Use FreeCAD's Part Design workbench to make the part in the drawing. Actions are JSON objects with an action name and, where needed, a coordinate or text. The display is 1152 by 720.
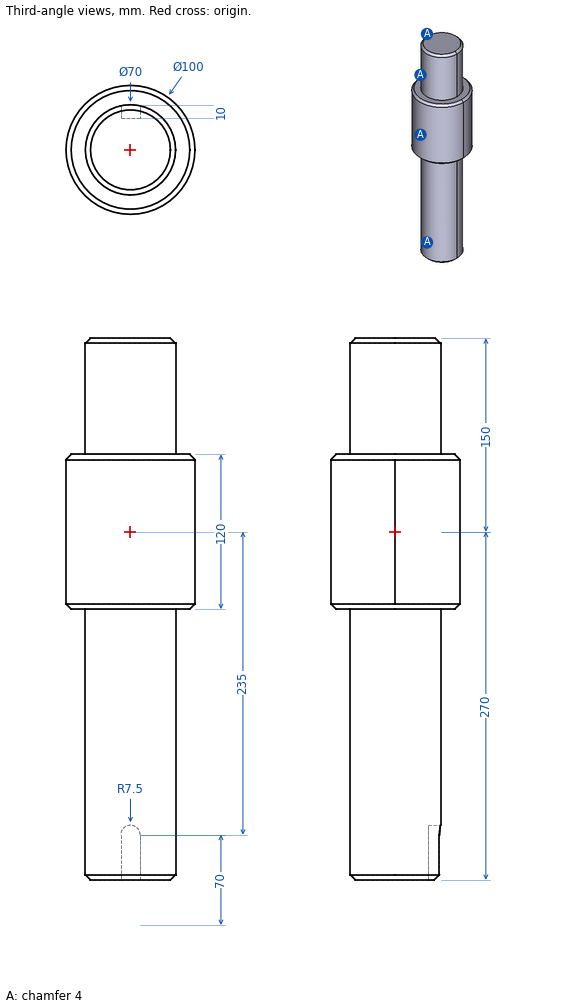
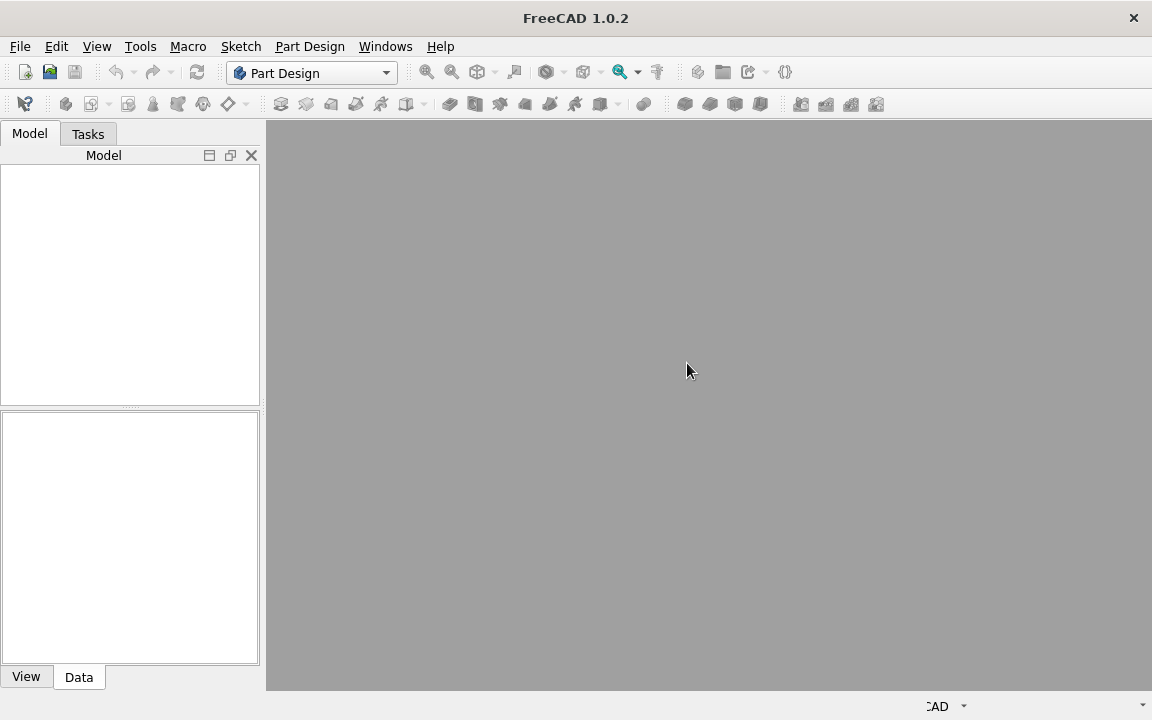
{"action": "left_click", "coordinate": [25, 72]}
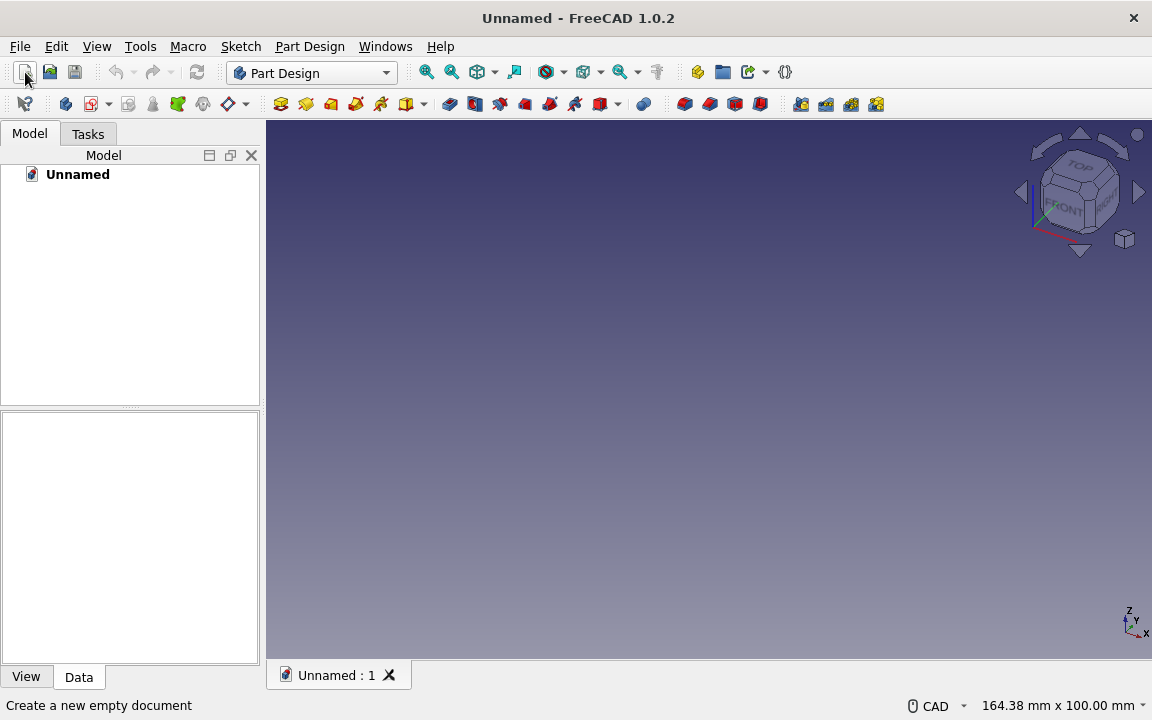
{"action": "left_click", "coordinate": [90, 104]}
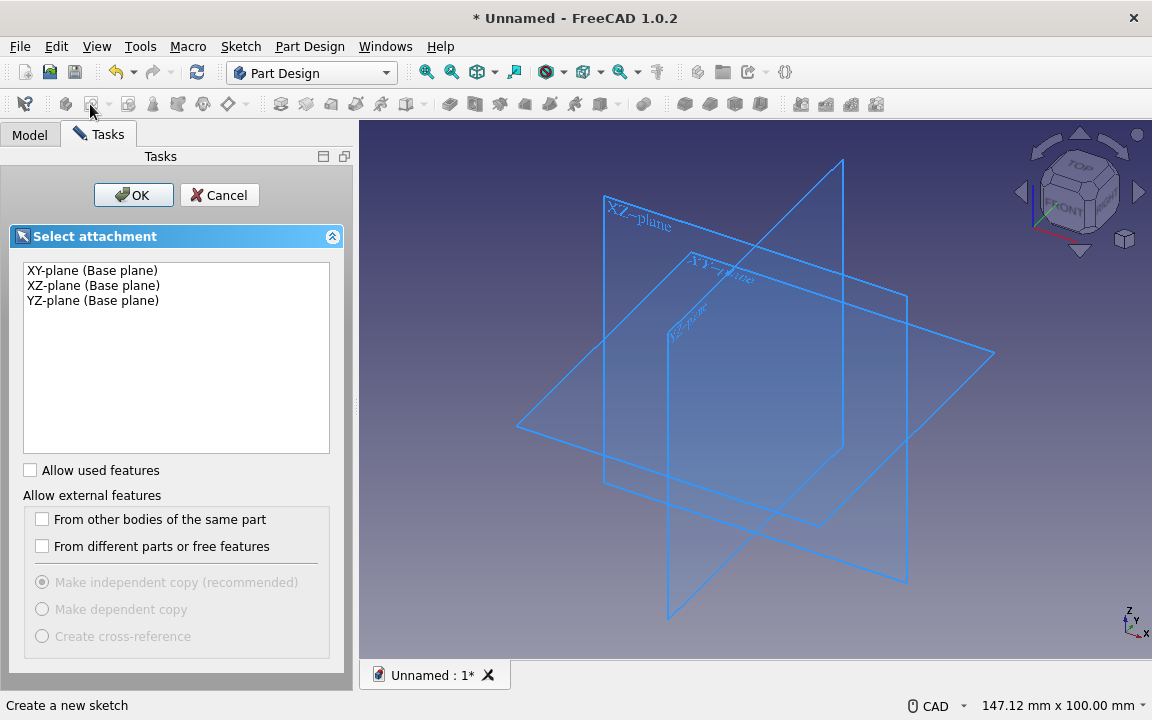
{"action": "left_click", "coordinate": [84, 270]}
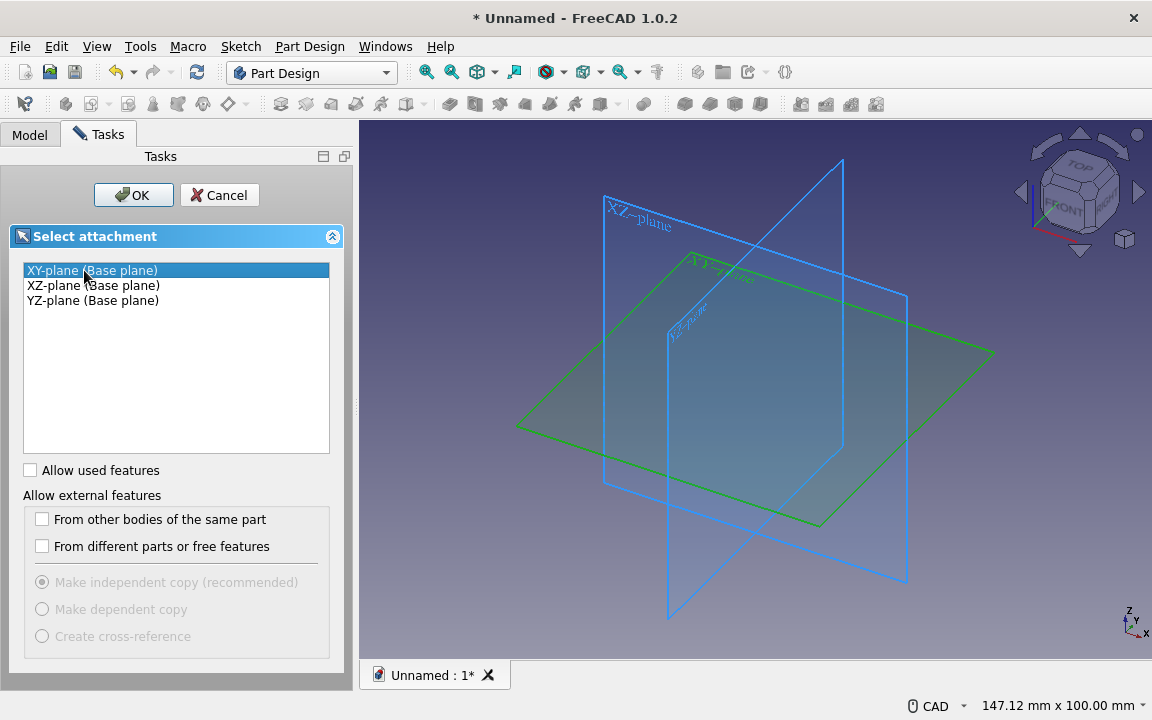
{"action": "left_click", "coordinate": [134, 195]}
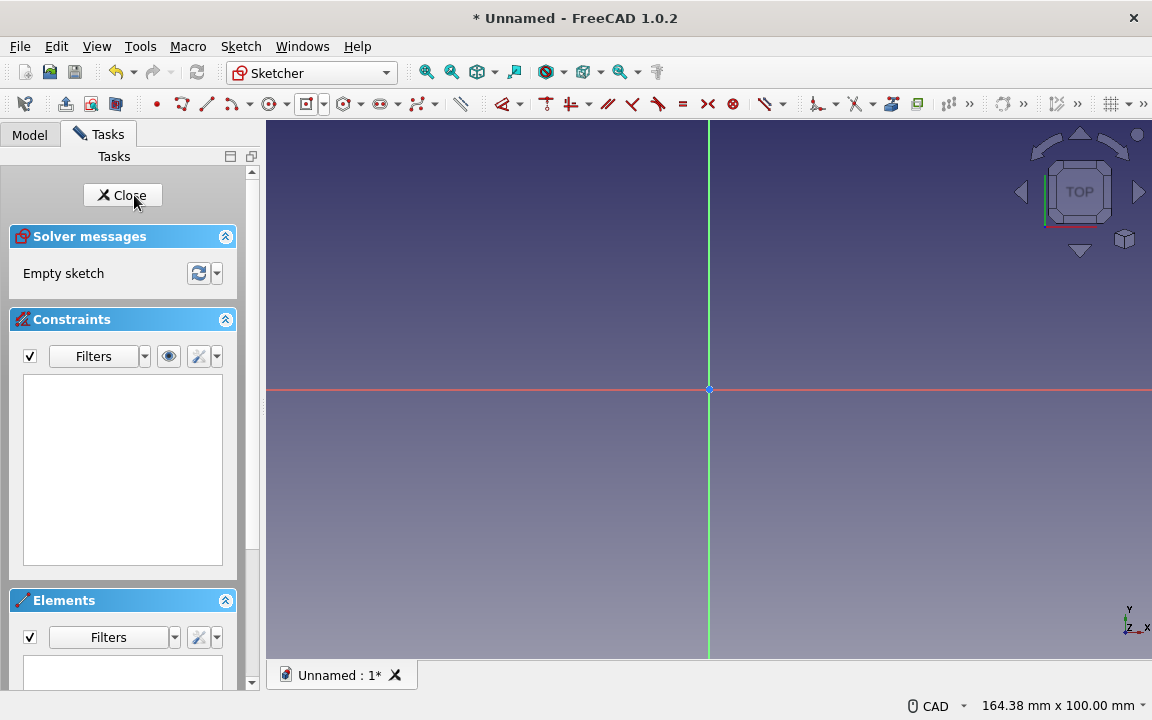
{"action": "left_click", "coordinate": [268, 104]}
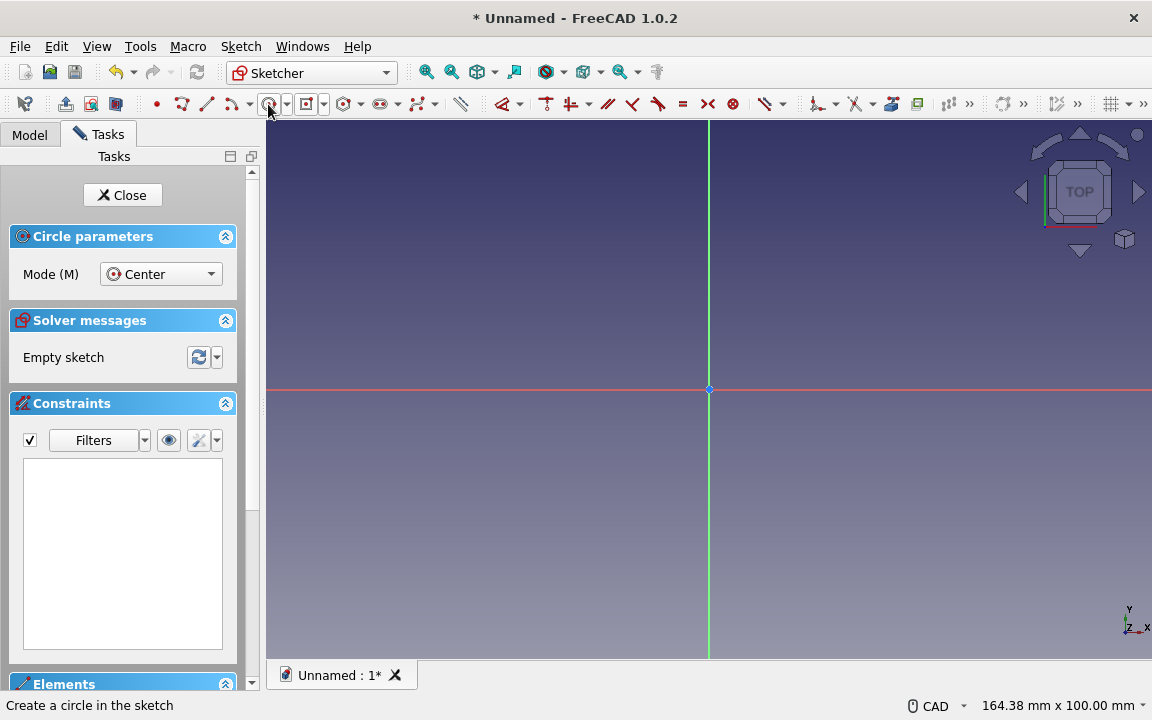
{"action": "left_click", "coordinate": [709, 390]}
{"action": "mouse_move", "coordinate": [842, 256]}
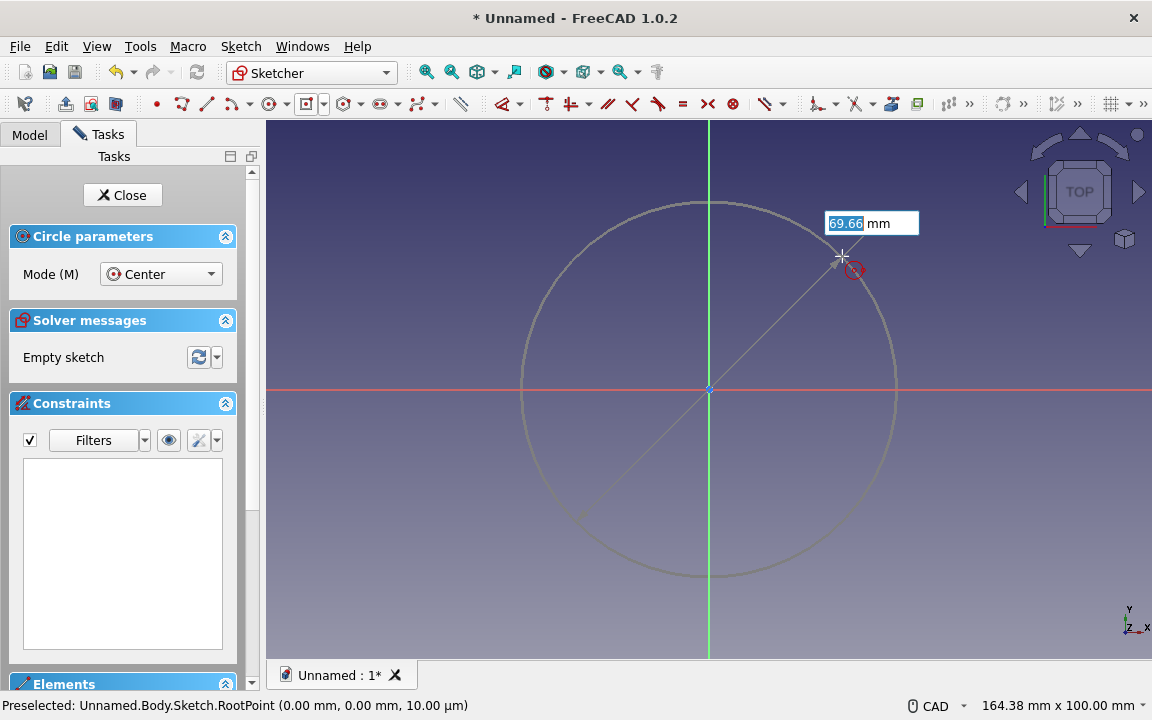
{"action": "type", "text": "70"}
{"action": "key", "text": "Return"}
{"action": "key", "text": "Escape"}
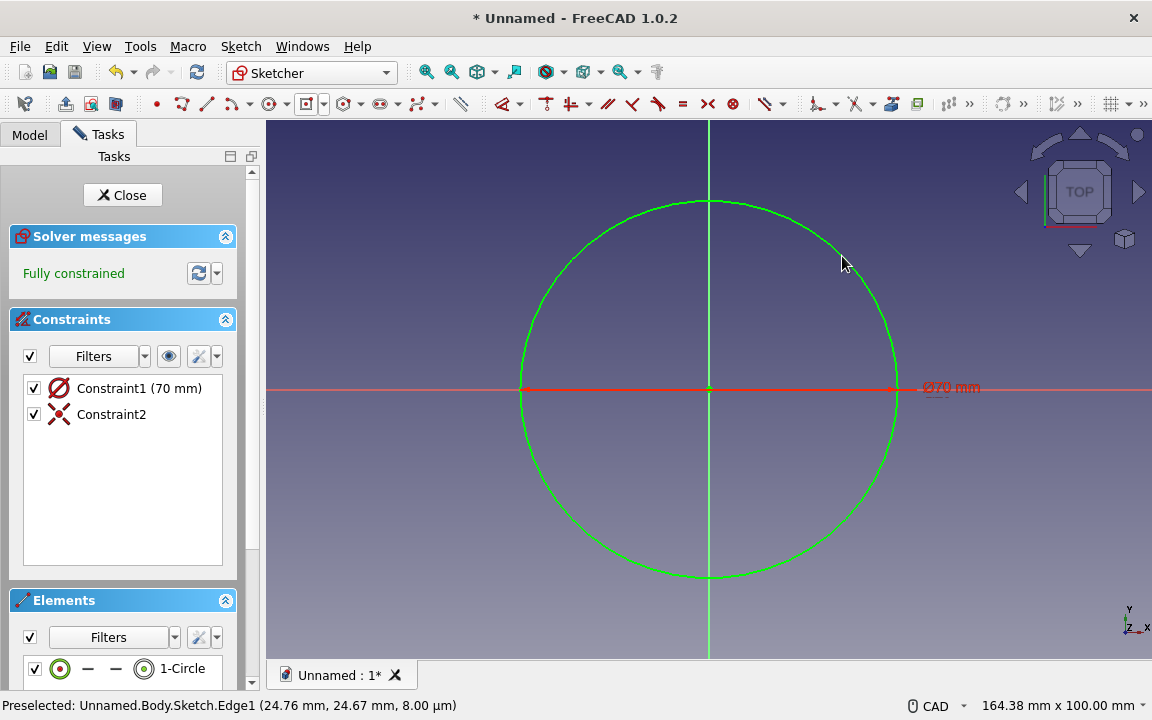
{"action": "left_click", "coordinate": [123, 195]}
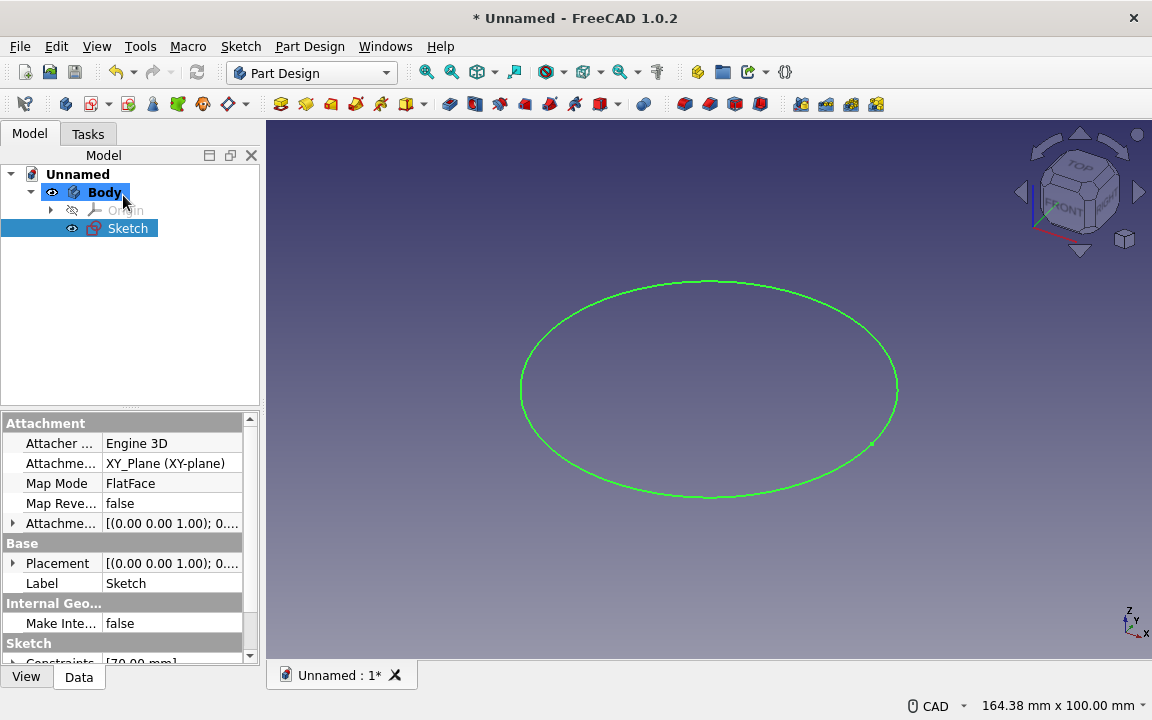
{"action": "left_click", "coordinate": [281, 104]}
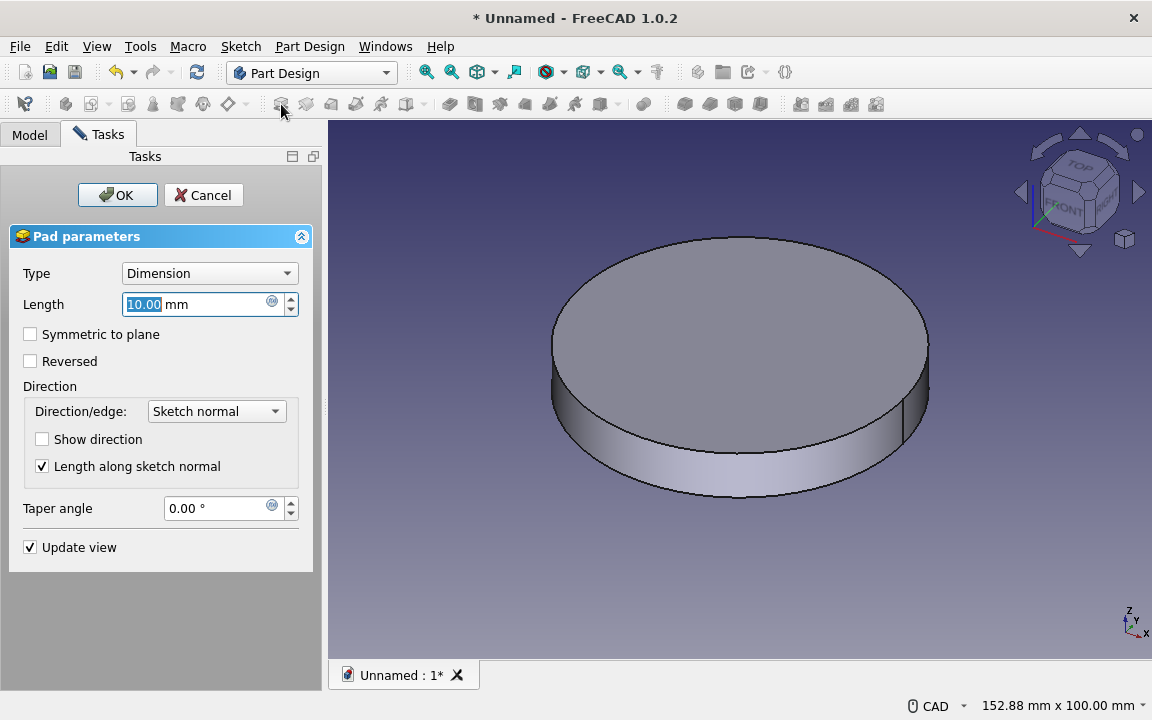
{"action": "left_click", "coordinate": [210, 274]}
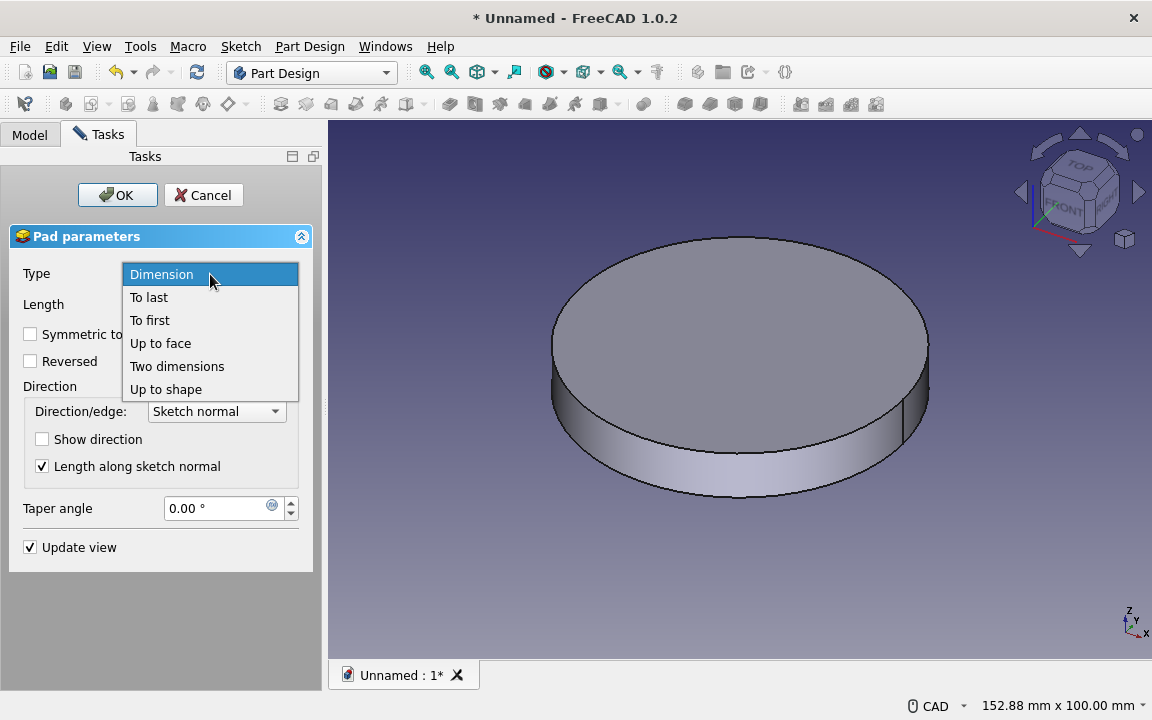
{"action": "left_click", "coordinate": [208, 366]}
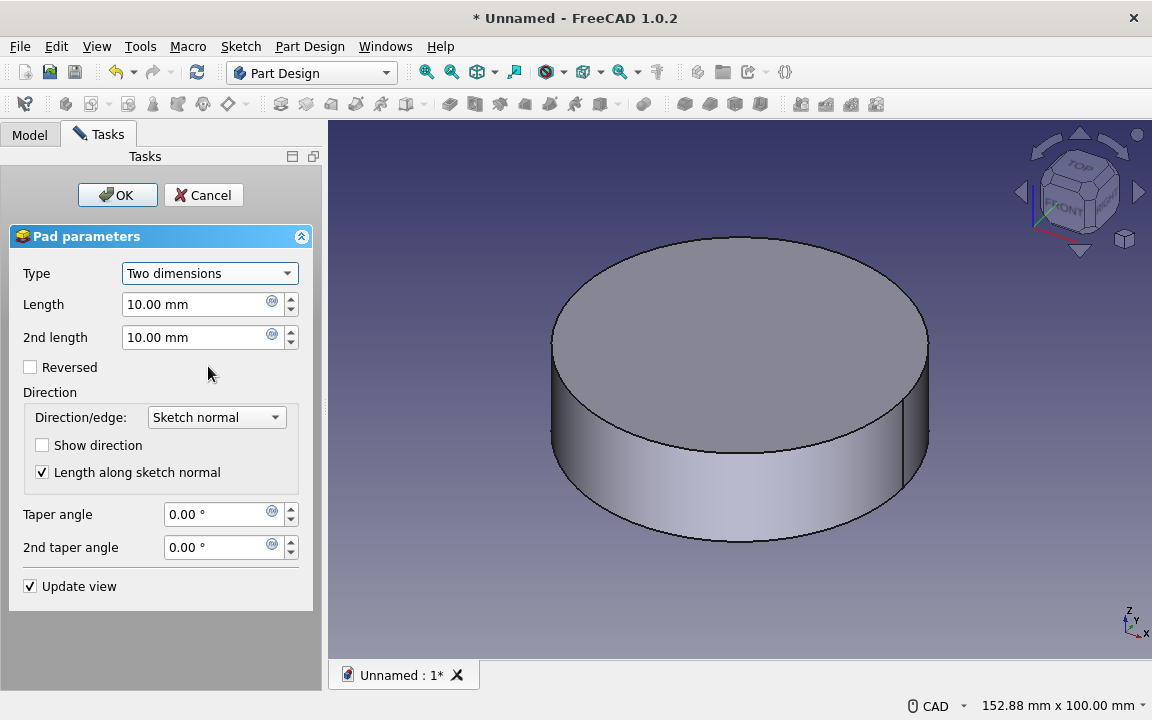
{"action": "triple_click", "coordinate": [204, 304]}